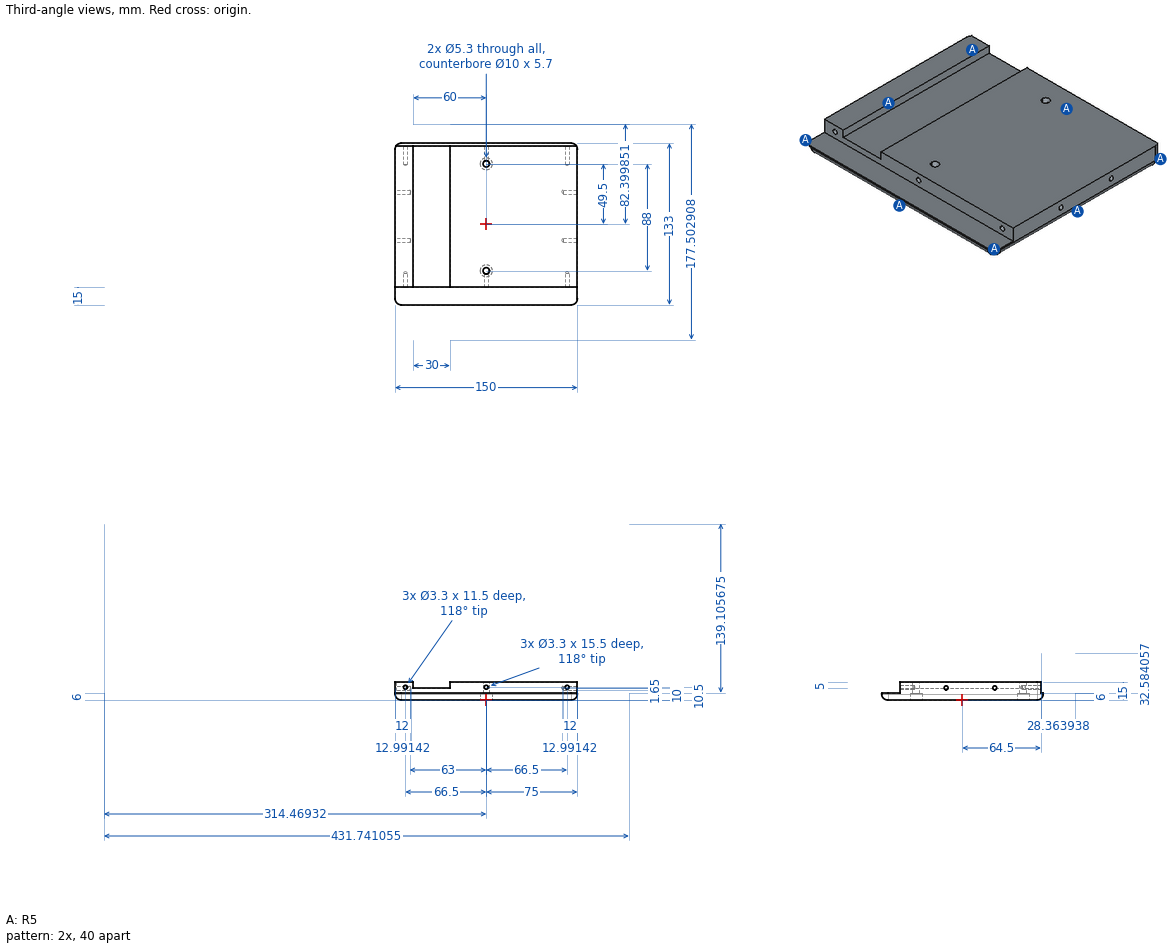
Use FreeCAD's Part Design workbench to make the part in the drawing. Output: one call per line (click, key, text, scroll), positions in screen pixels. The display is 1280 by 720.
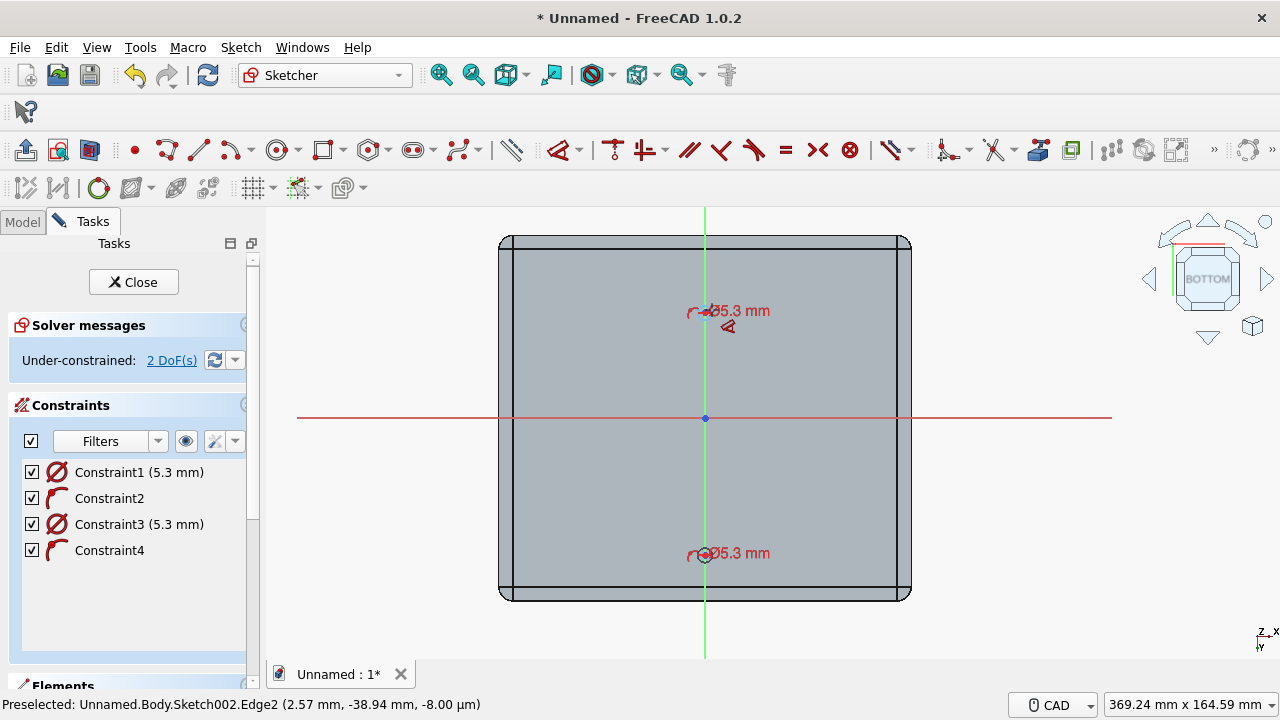
click(705, 555)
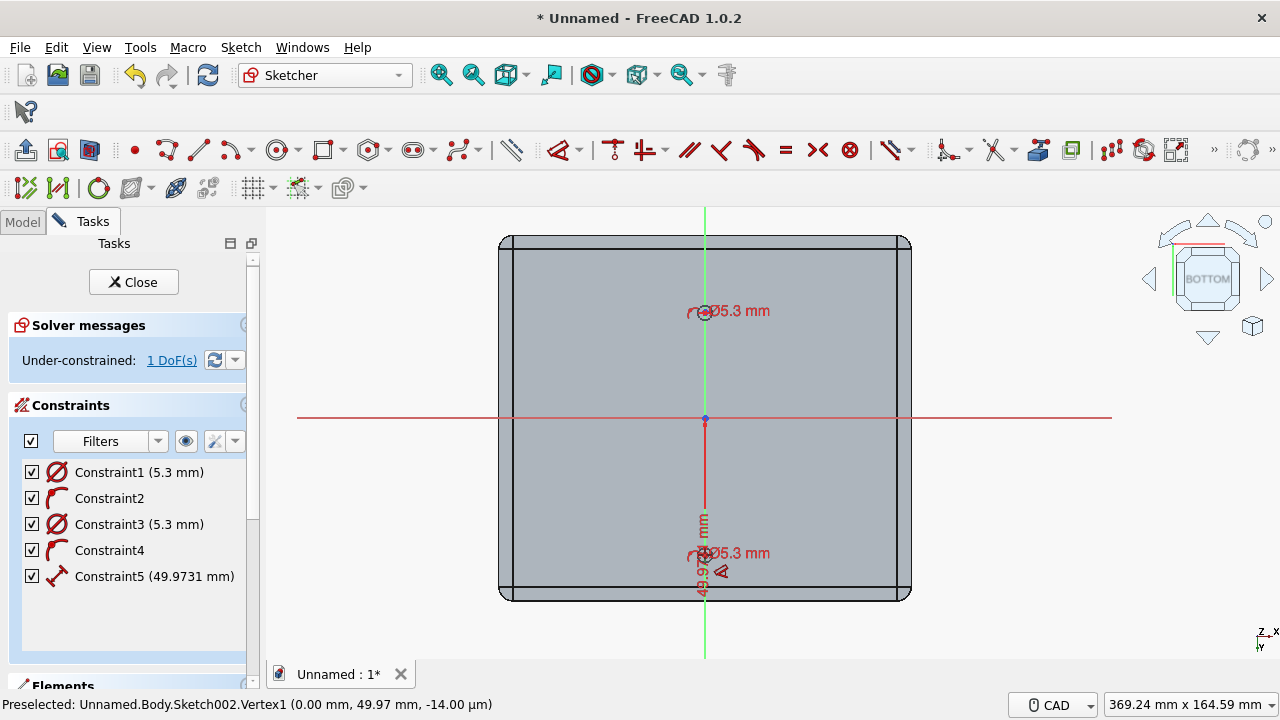
click(705, 313)
click(739, 434)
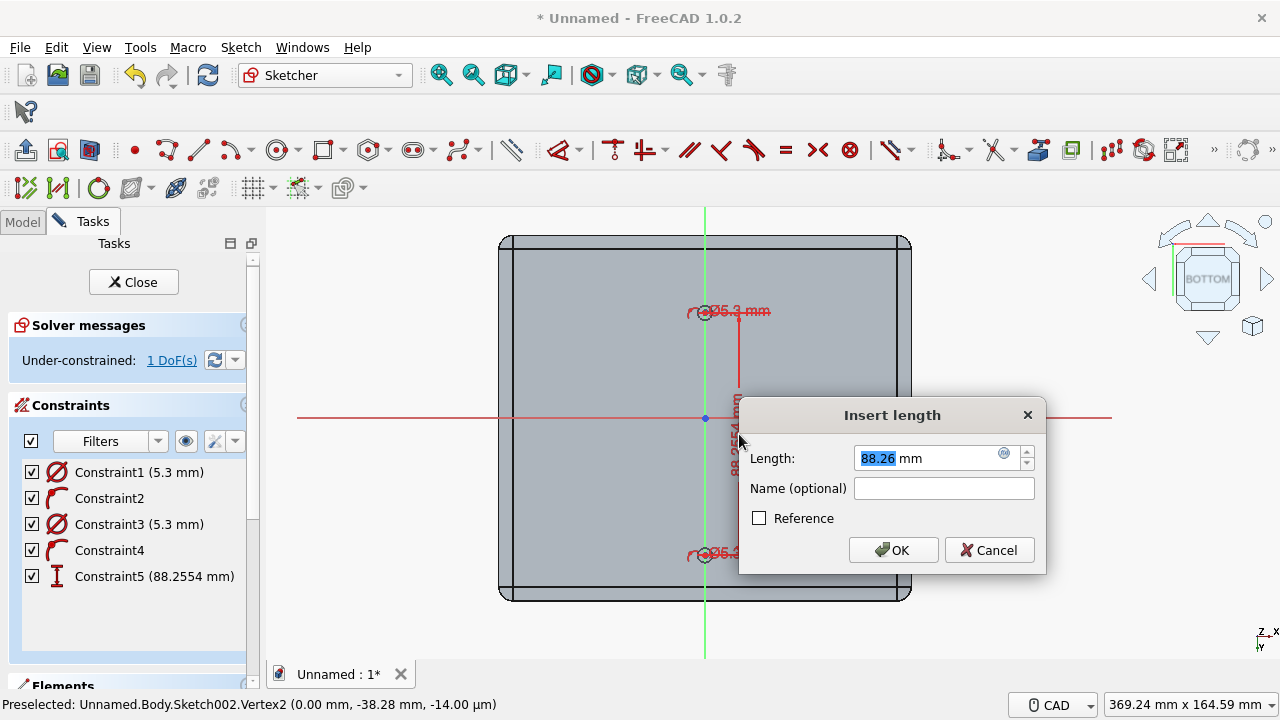
text(88)
key(Return)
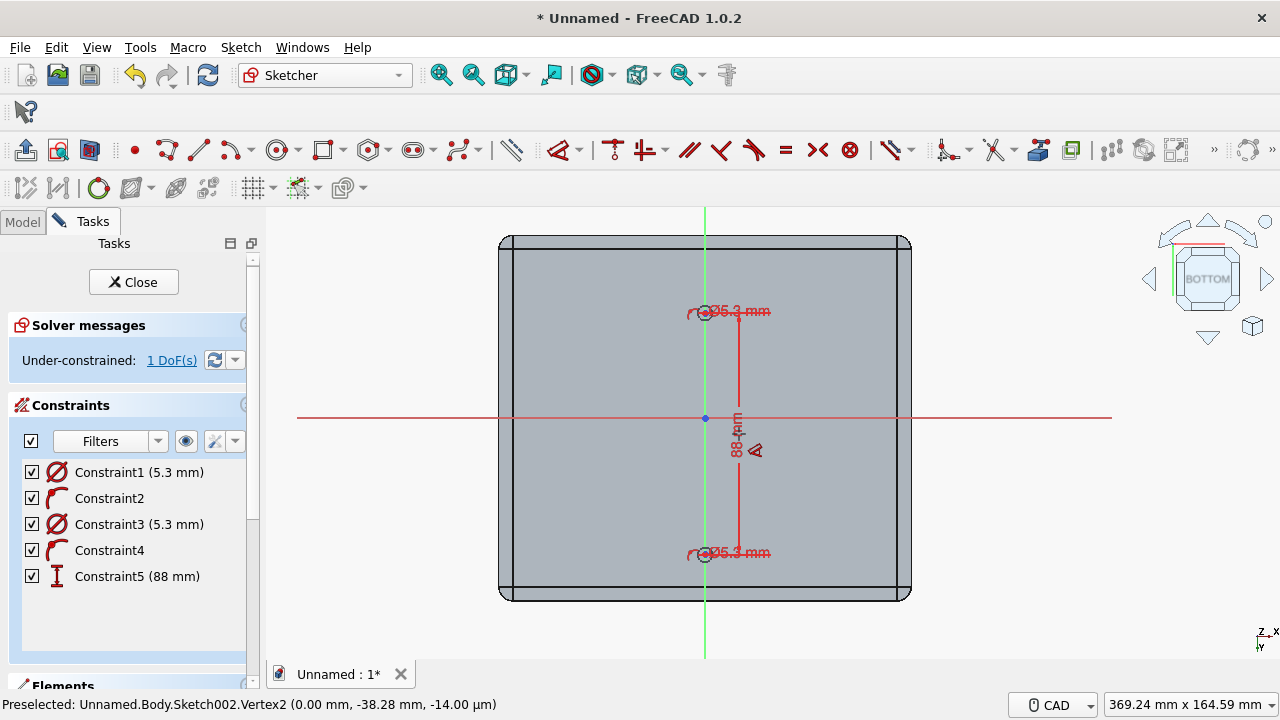
click(705, 555)
click(739, 486)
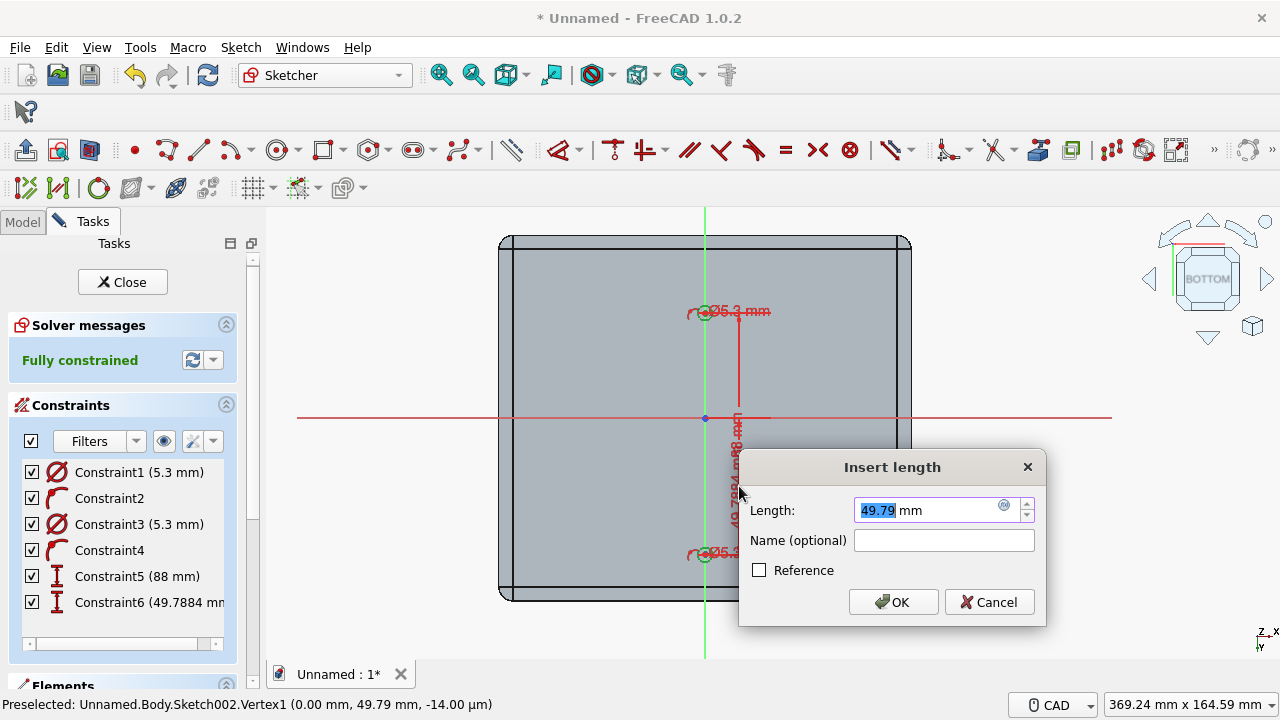
text(49.5)
key(Return)
key(Escape)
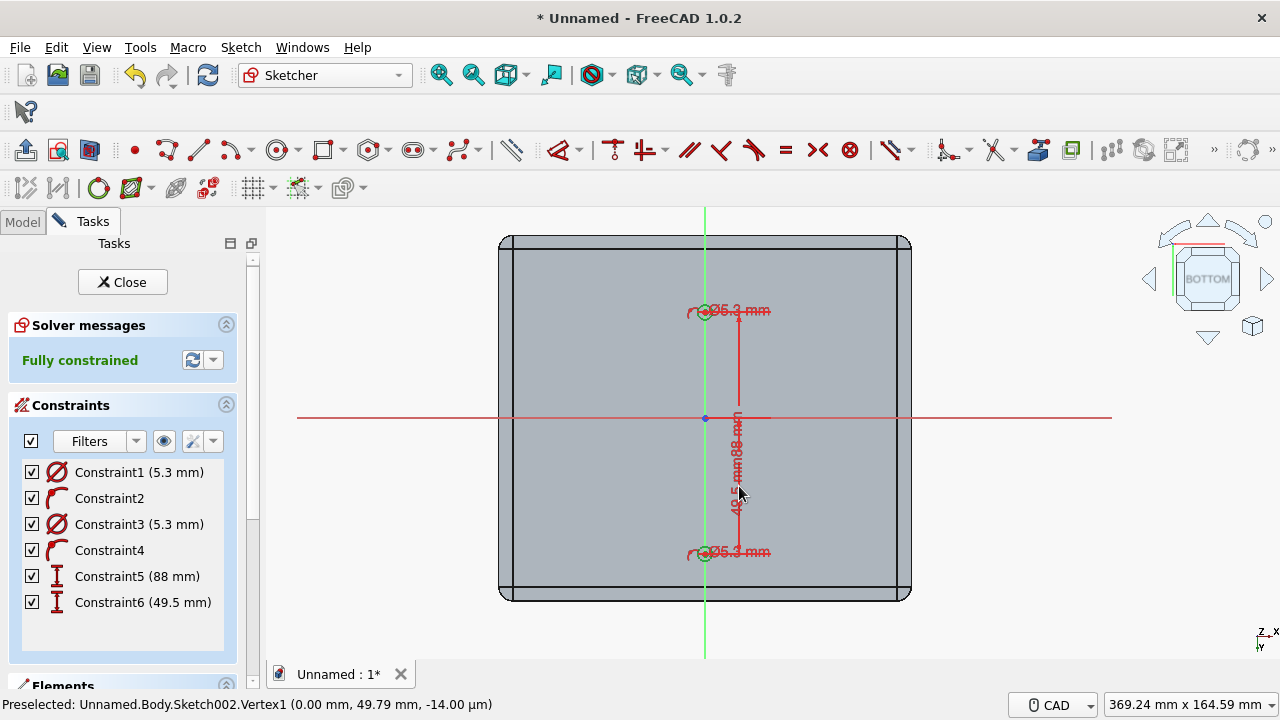
click(123, 282)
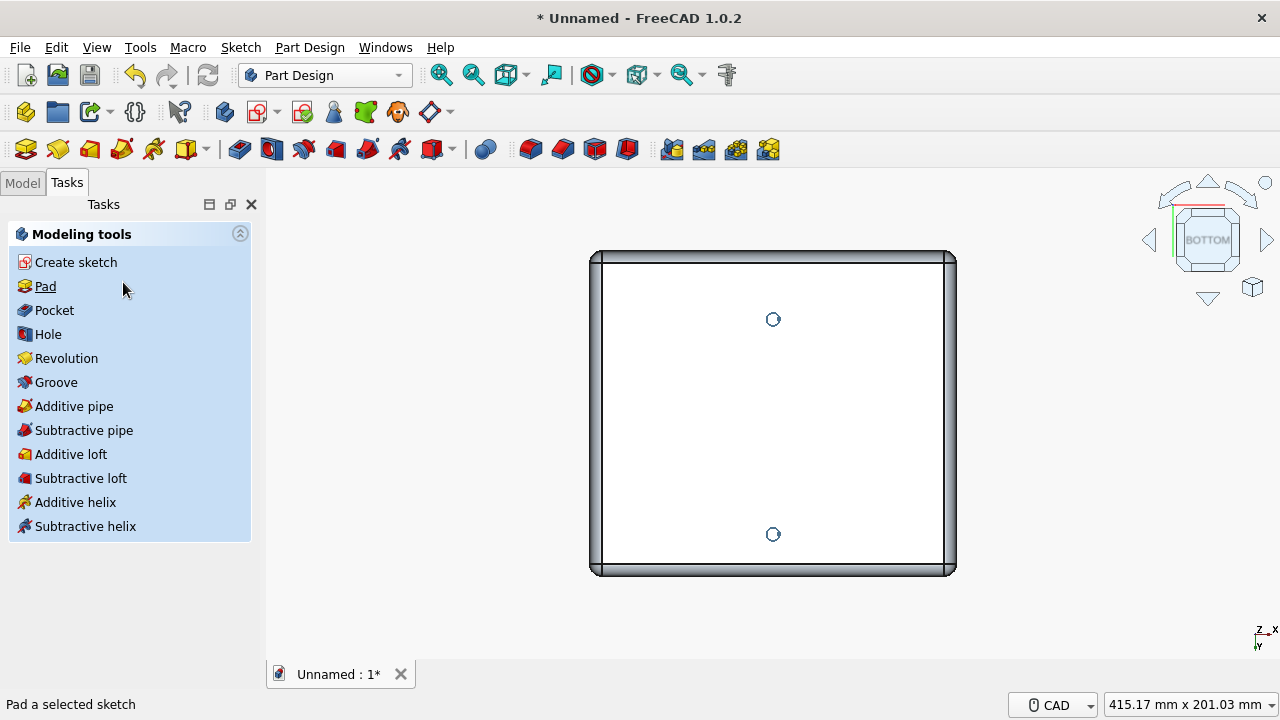
click(272, 150)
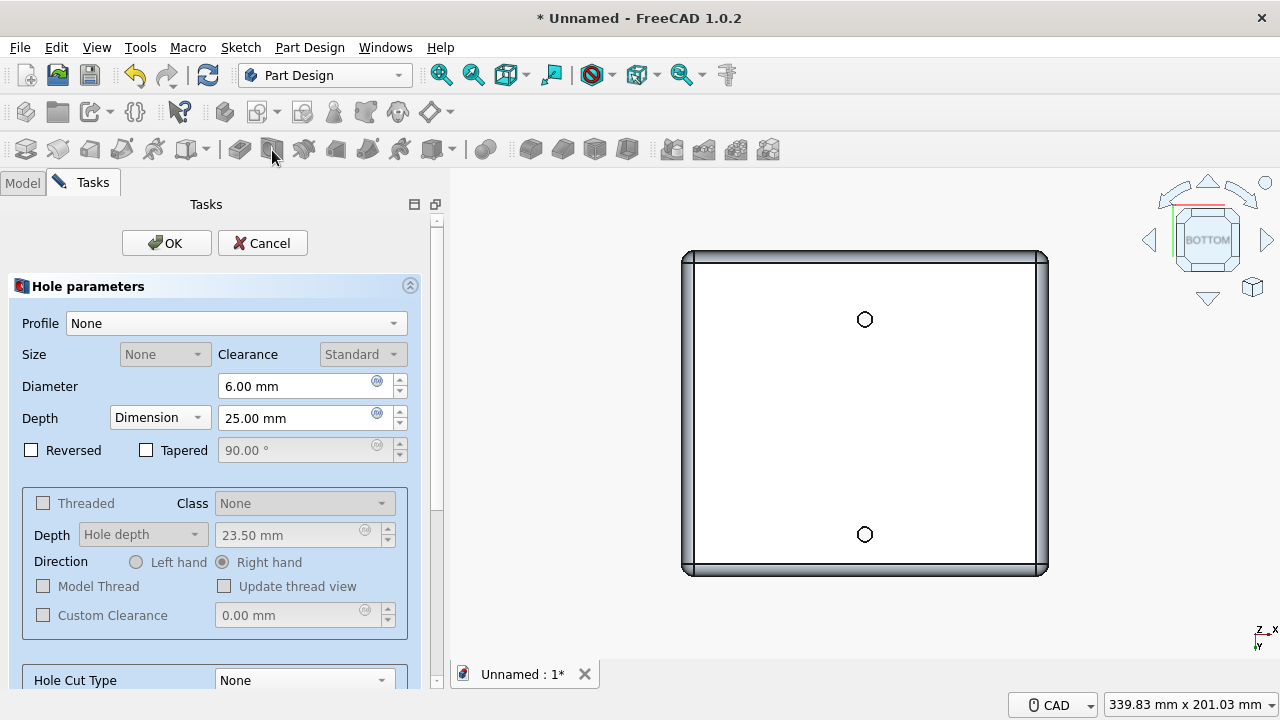
triple_click(305, 386)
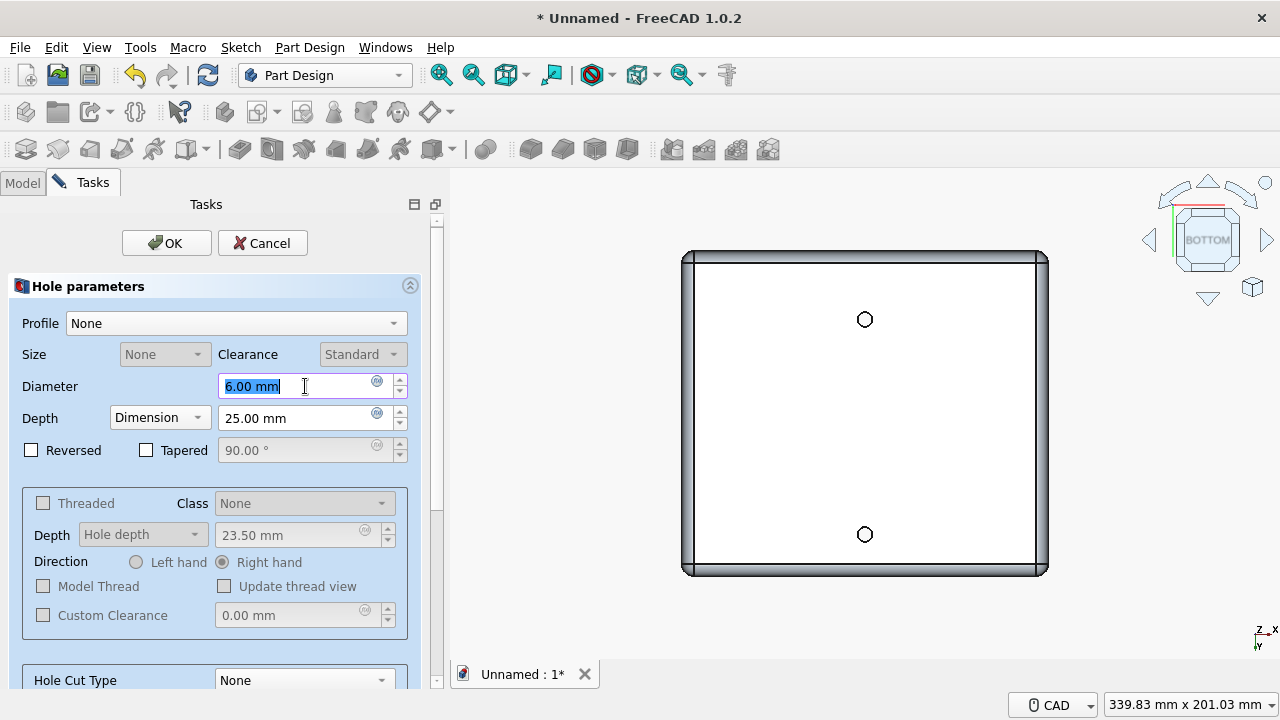
text(5.3)
key(Tab)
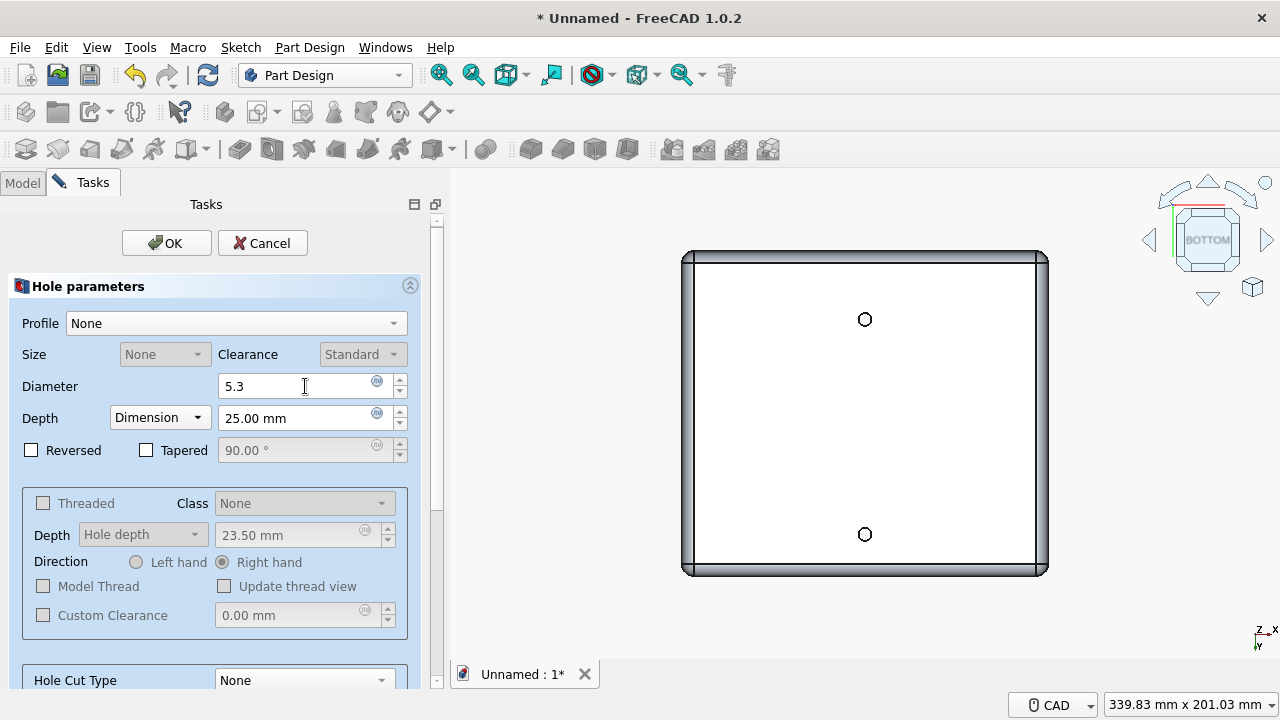
click(161, 418)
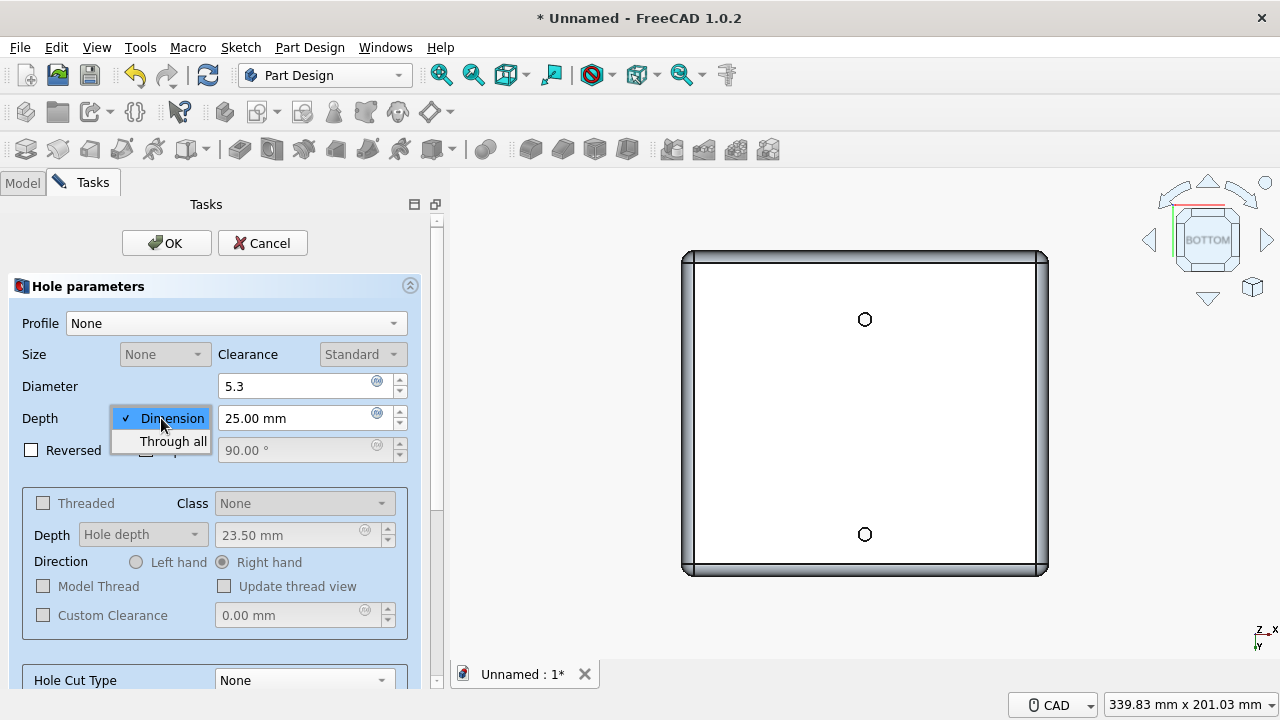
click(160, 442)